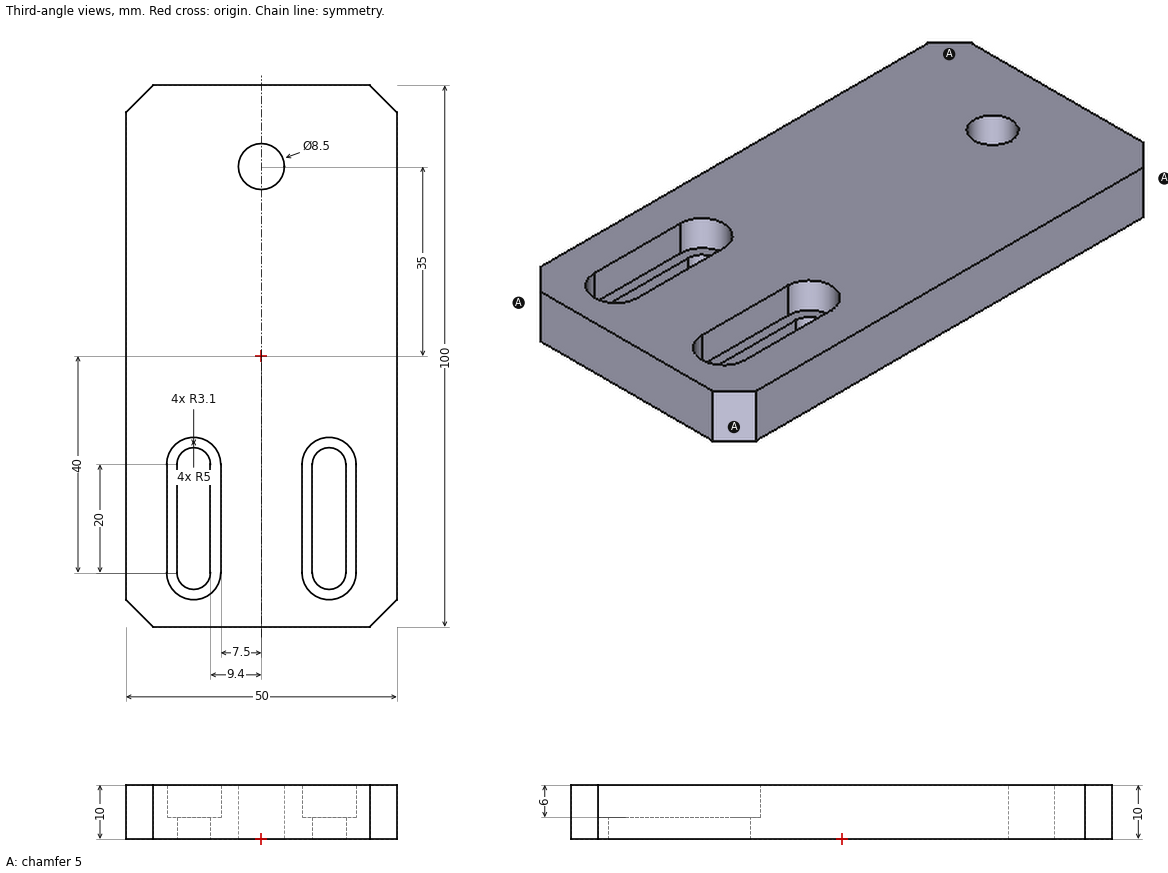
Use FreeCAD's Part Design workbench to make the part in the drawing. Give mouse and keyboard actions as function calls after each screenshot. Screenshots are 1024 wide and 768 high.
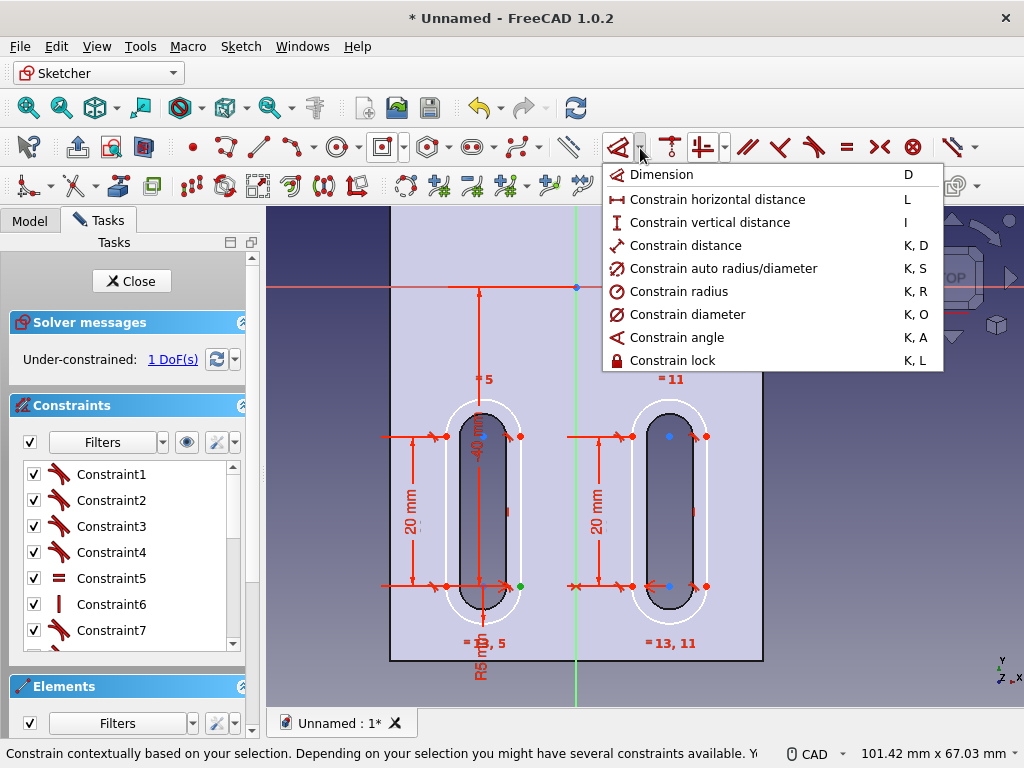
click(773, 200)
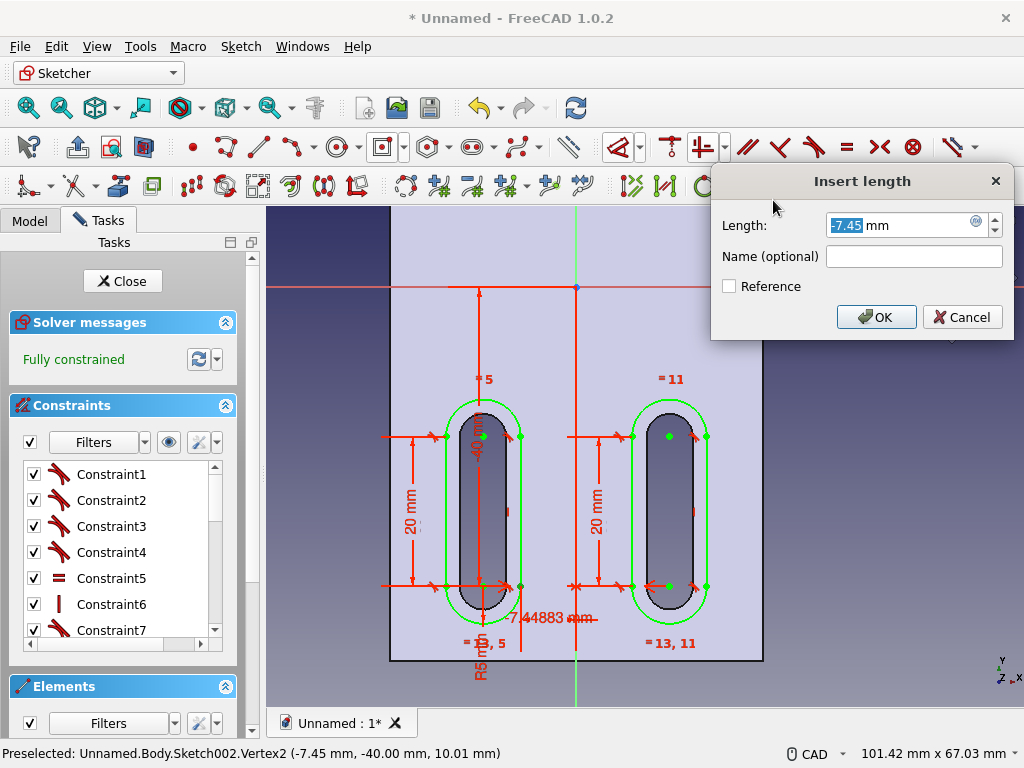
text(-7.5)
key(Return)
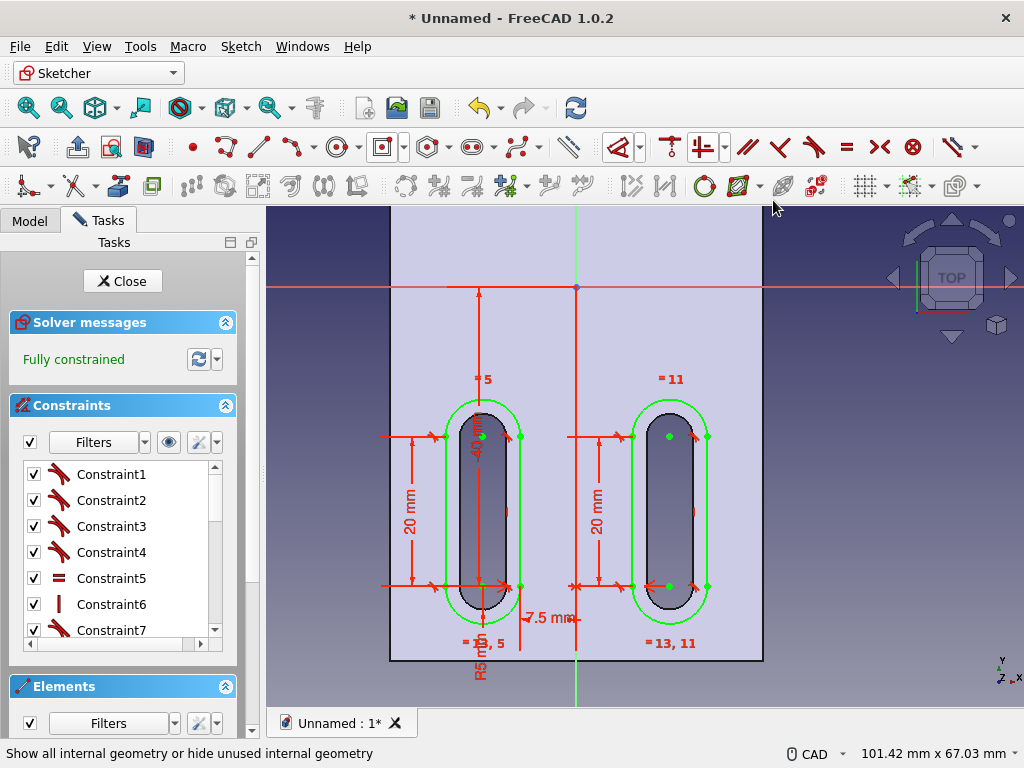
click(123, 281)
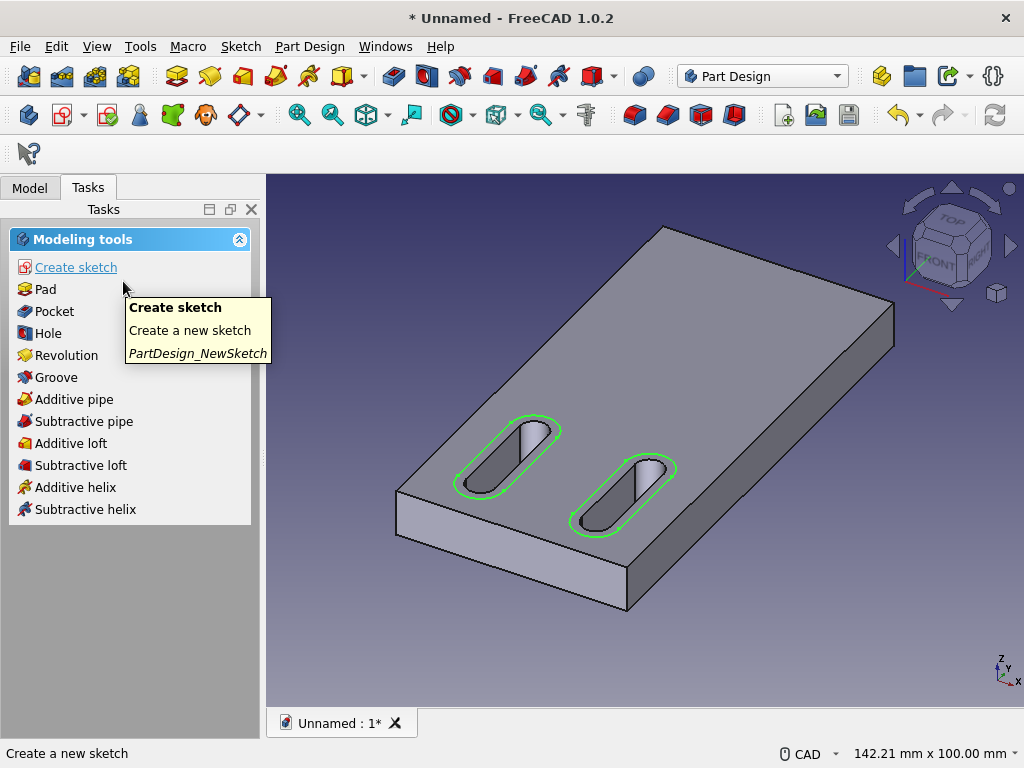
click(394, 76)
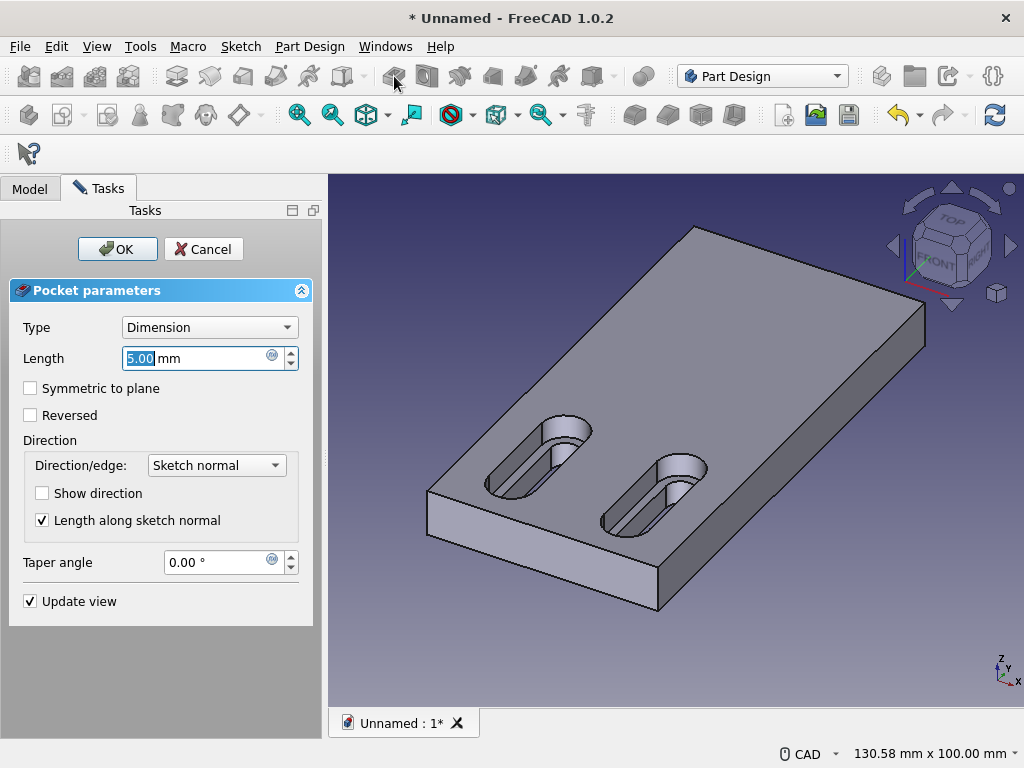
text(6)
key(Tab)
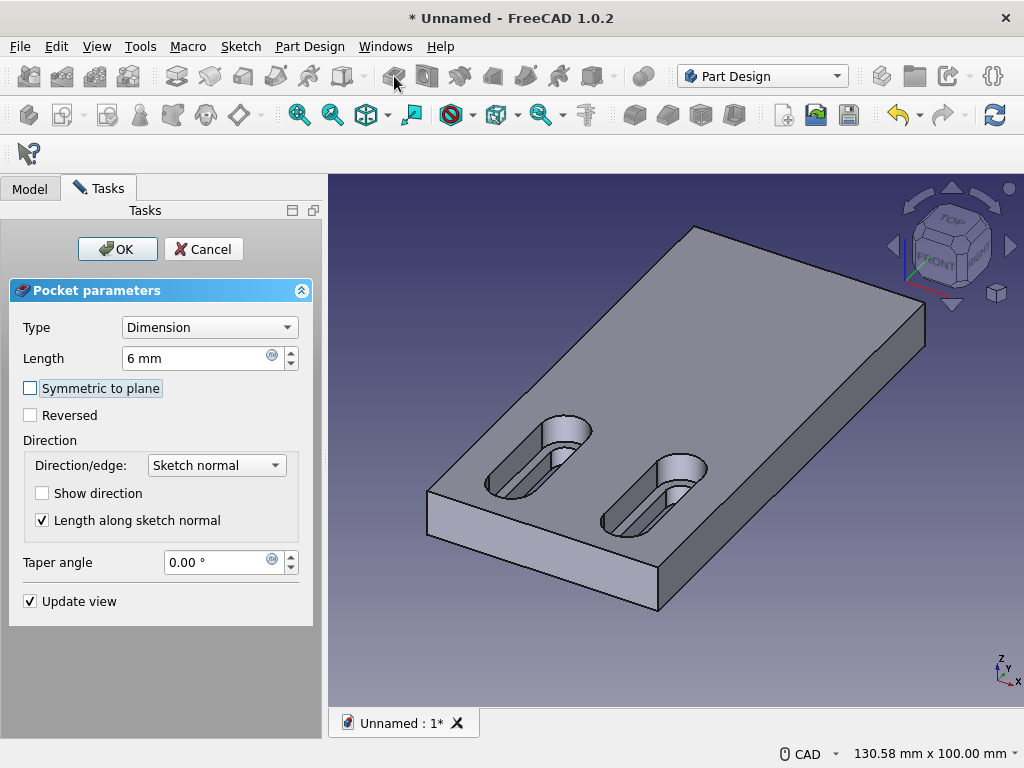
click(118, 249)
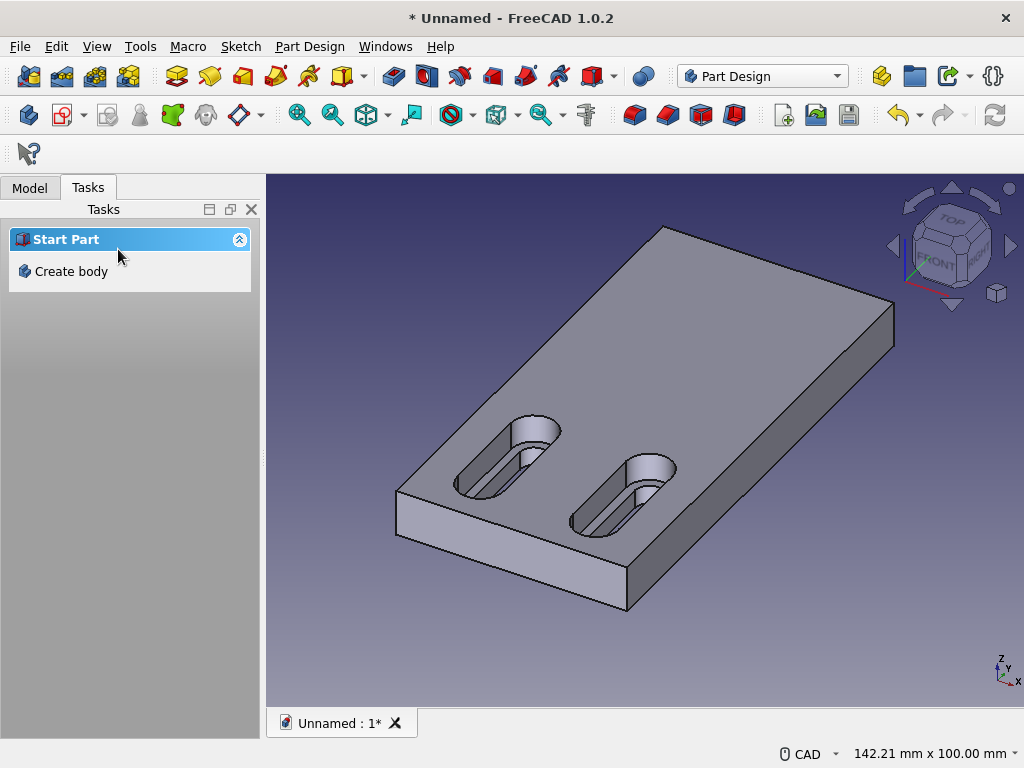
click(627, 588)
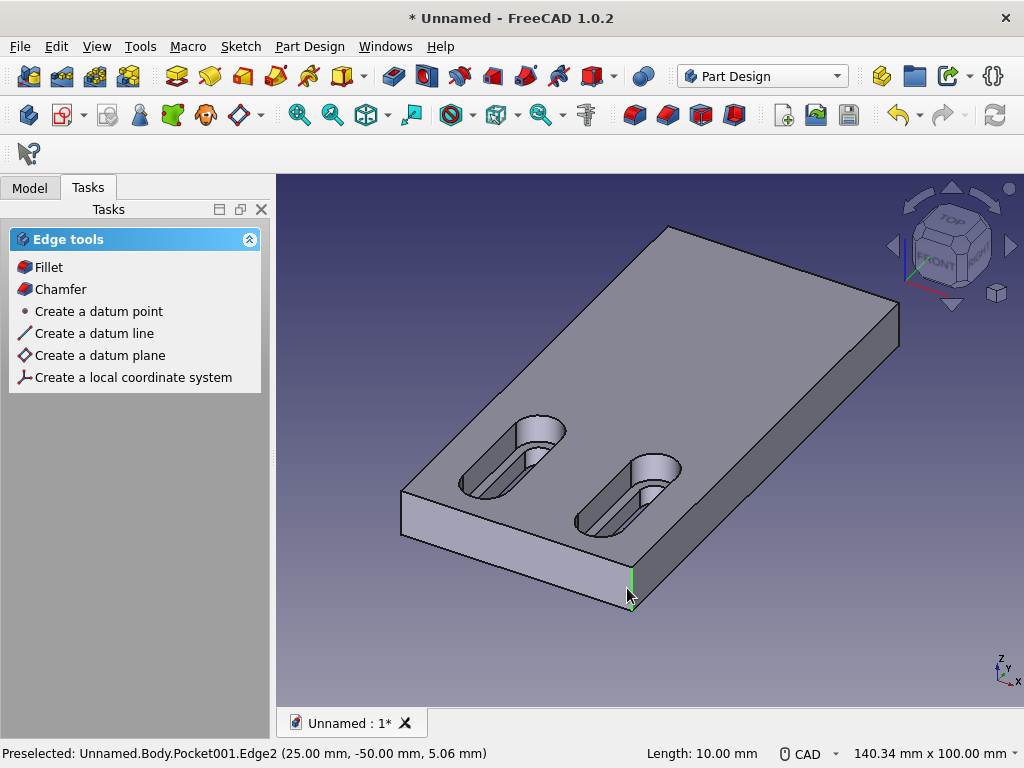
key(0)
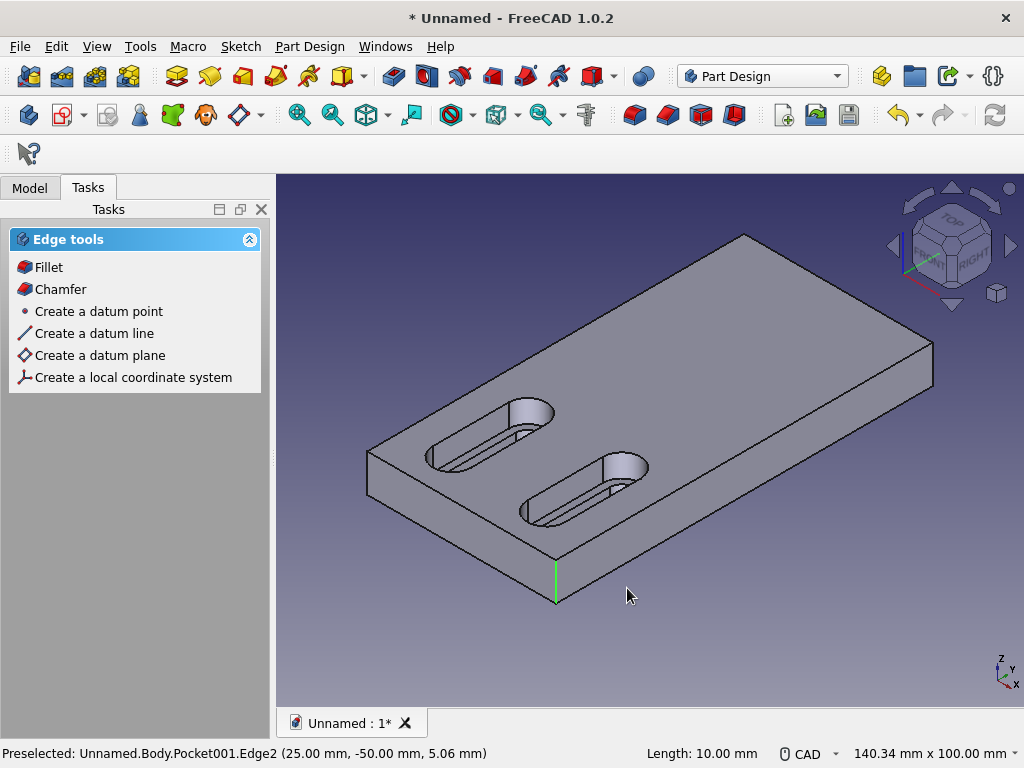
key(2)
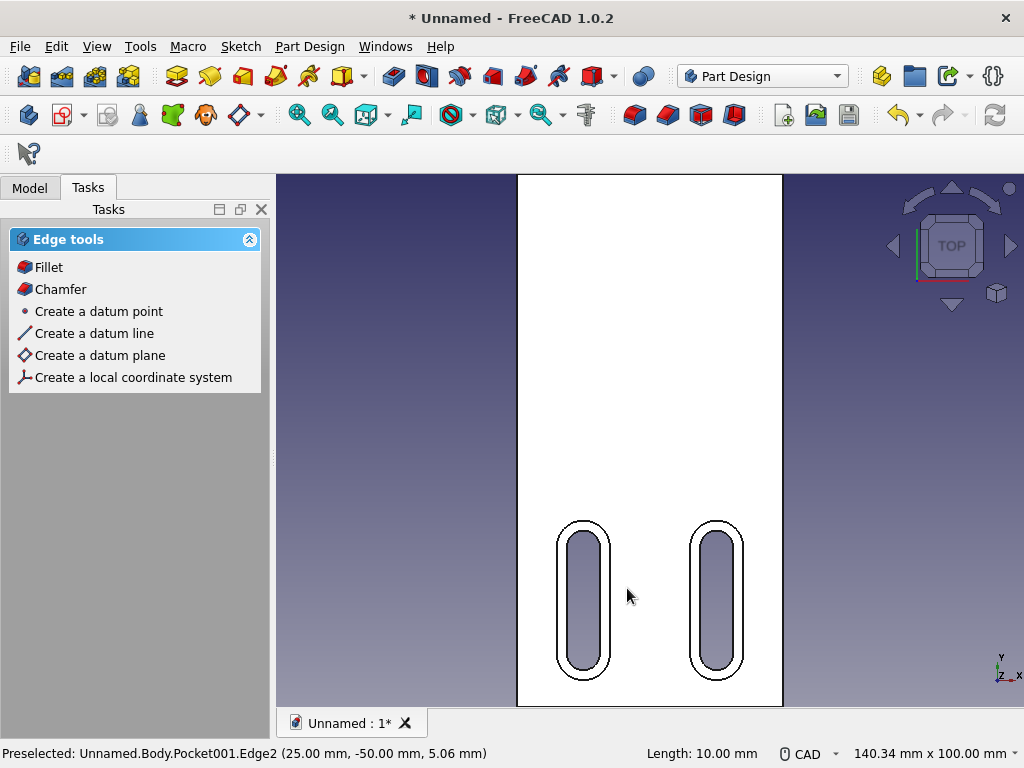
click(300, 116)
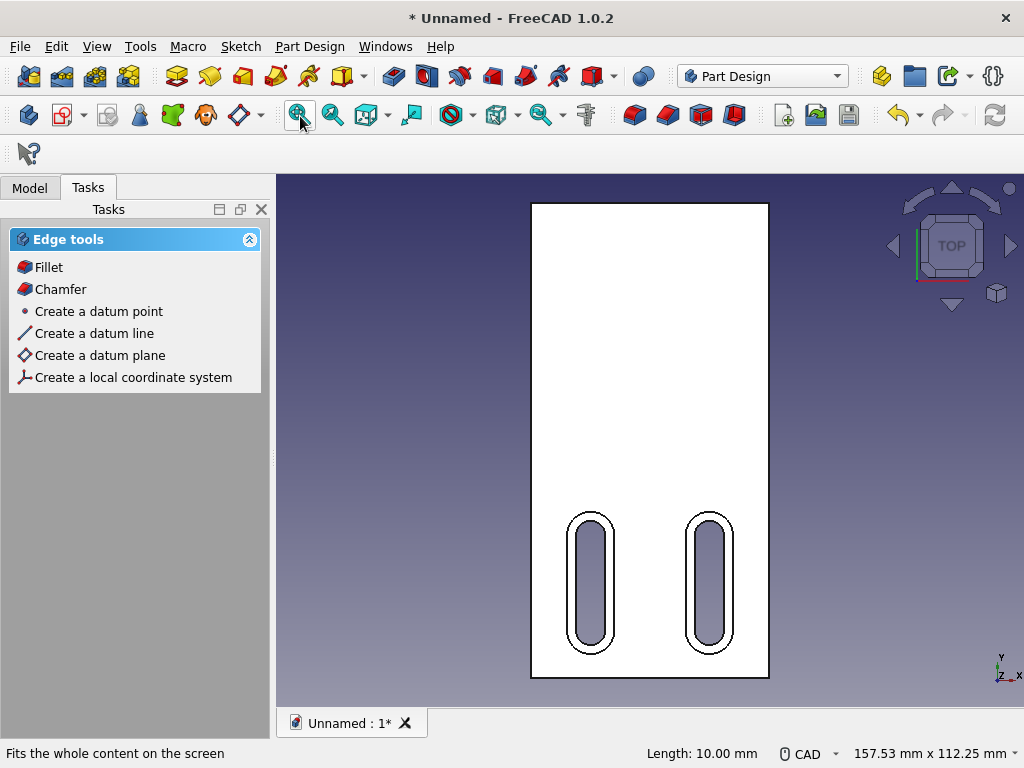
key(1)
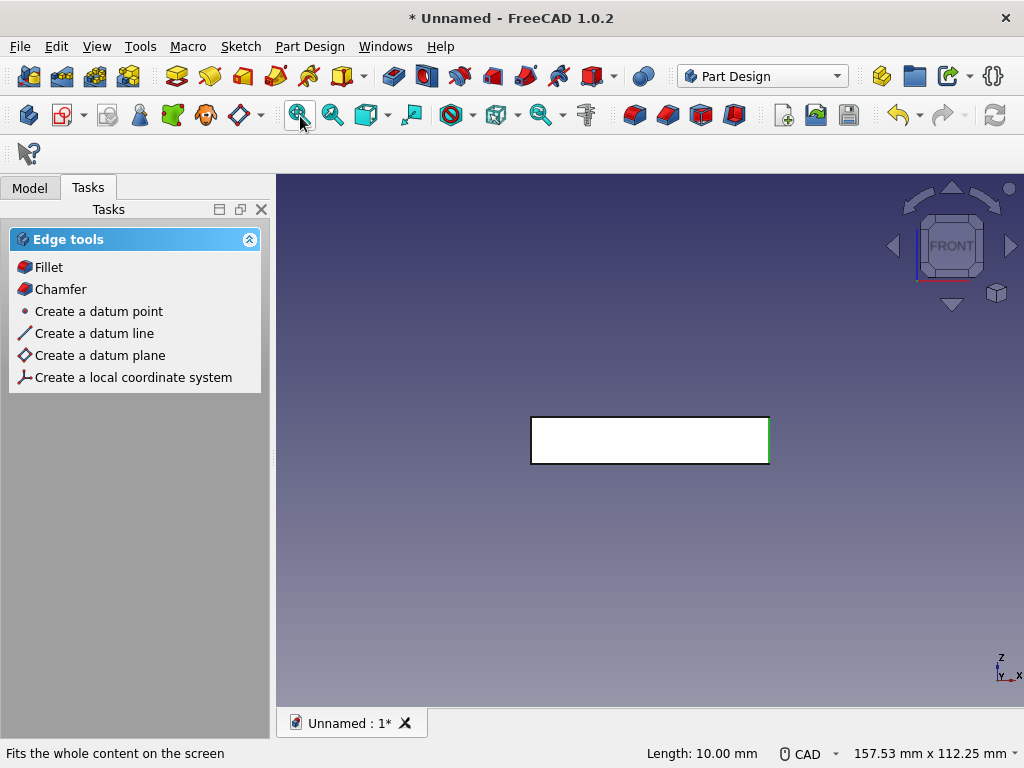
click(300, 116)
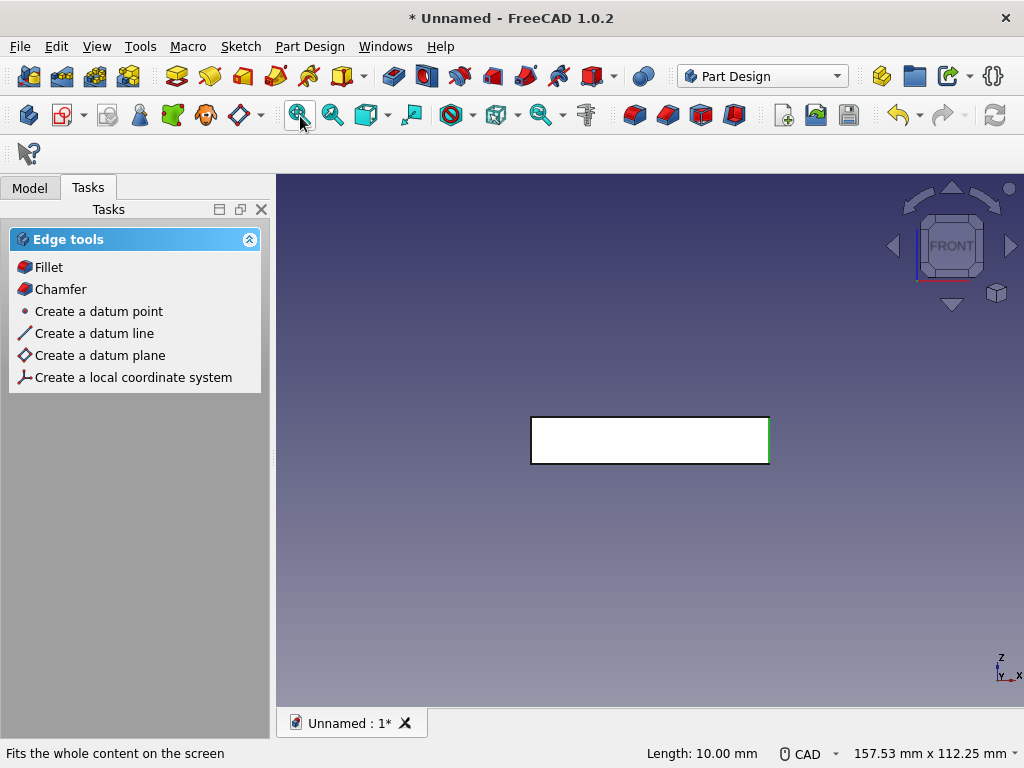
click(531, 440, ctrl)